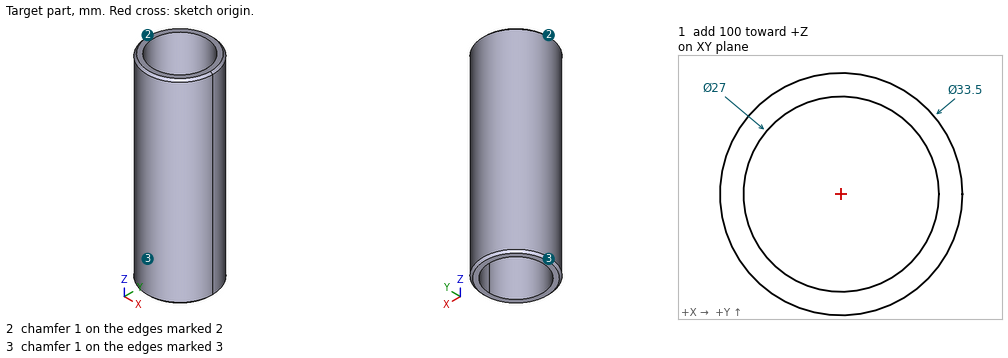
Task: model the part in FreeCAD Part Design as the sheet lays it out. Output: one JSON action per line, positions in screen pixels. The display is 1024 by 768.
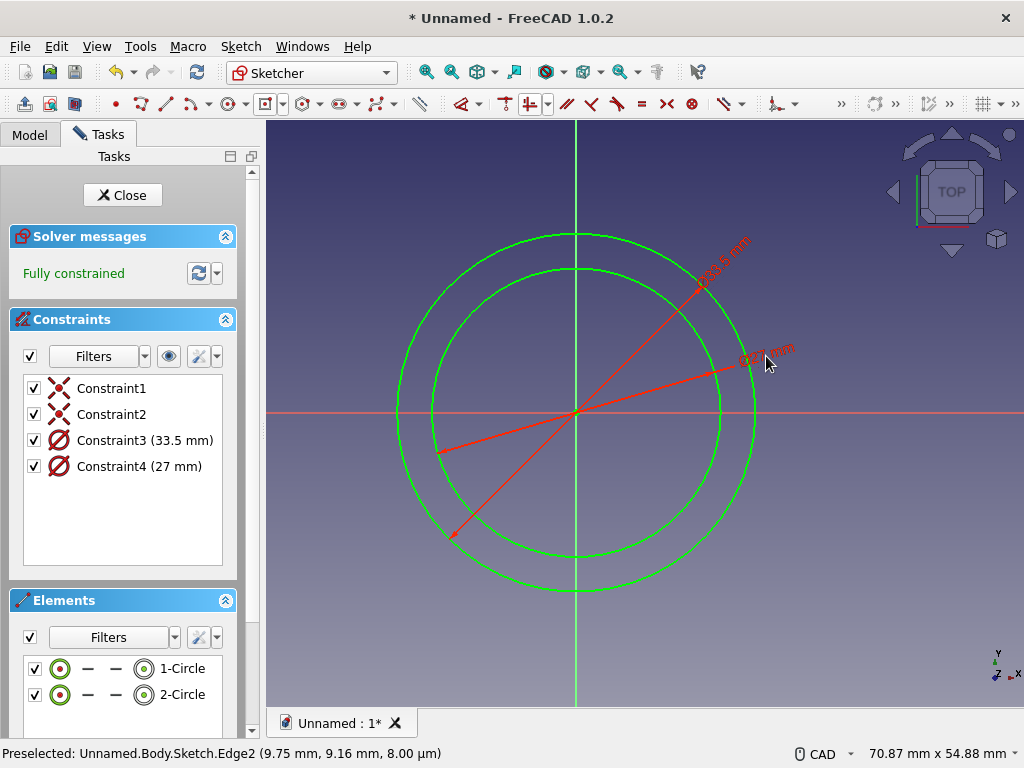
{"action": "left_click", "coordinate": [123, 195]}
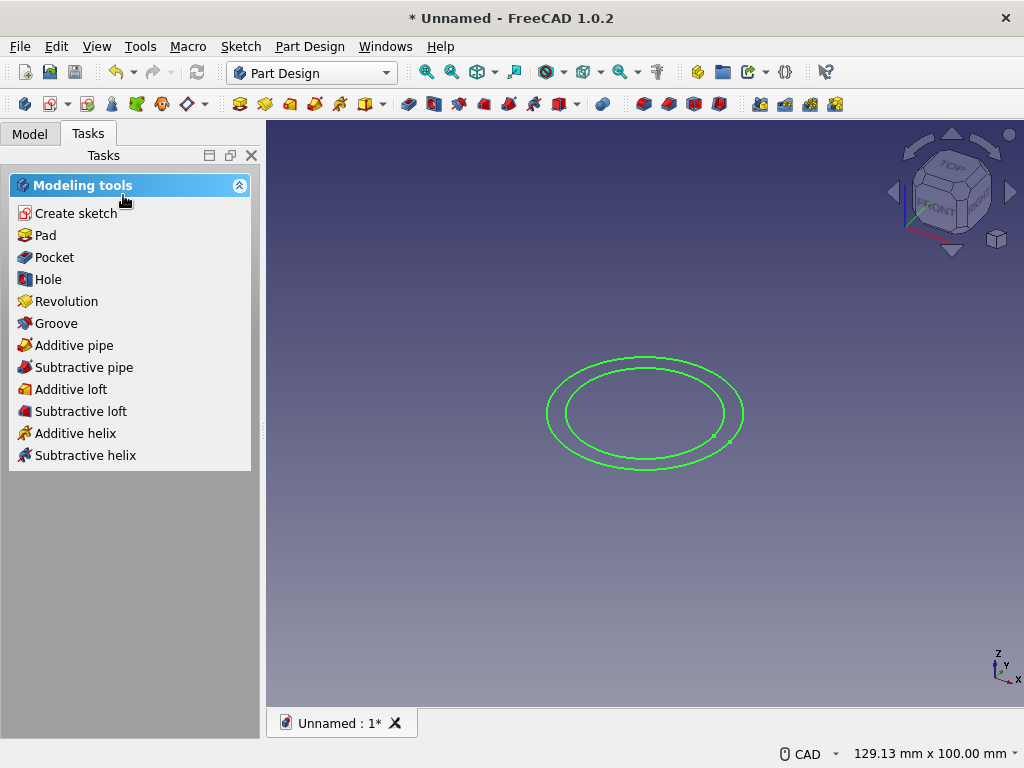
{"action": "left_click", "coordinate": [240, 104]}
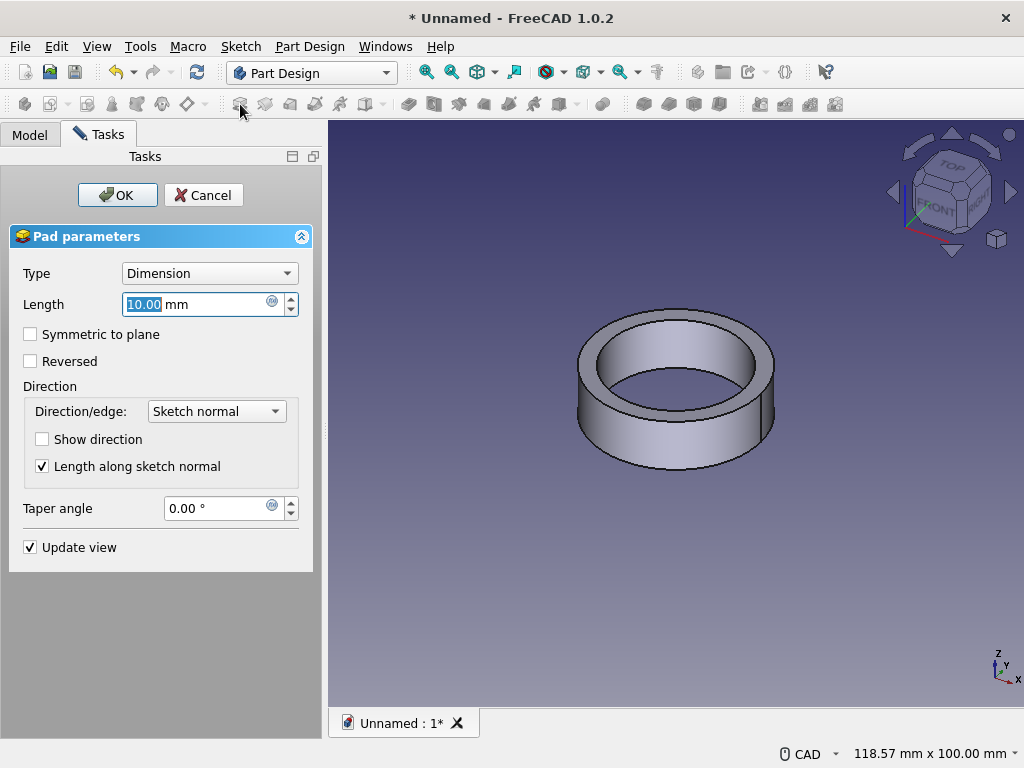
{"action": "type", "text": "100"}
{"action": "key", "text": "Tab"}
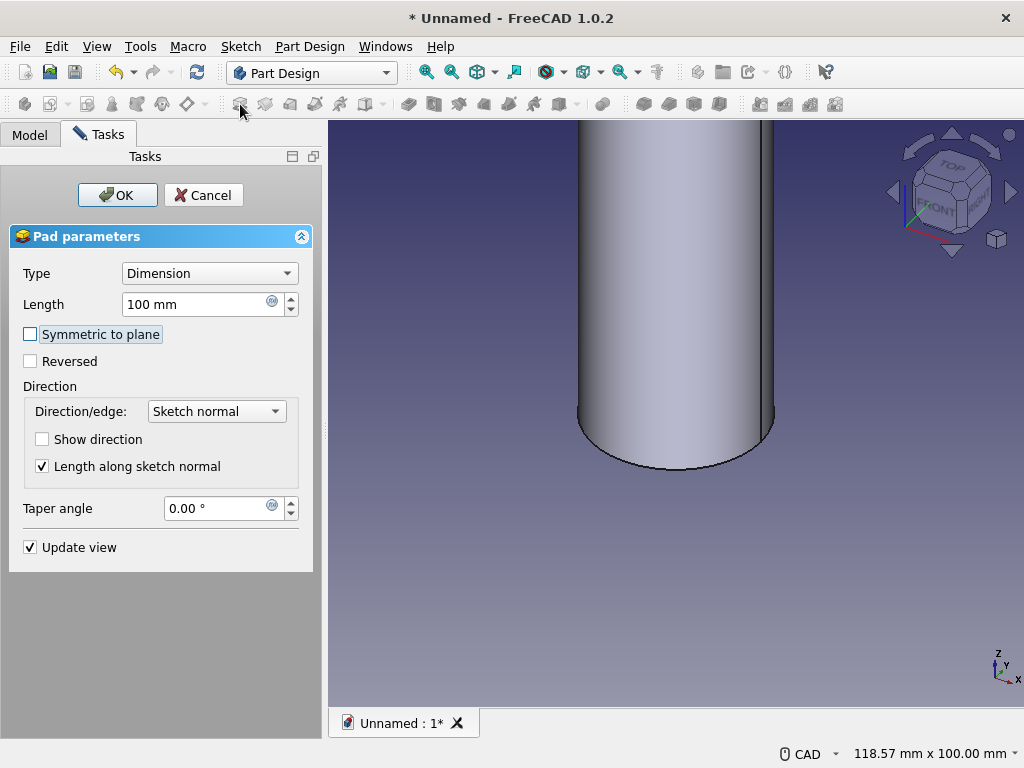
{"action": "left_click", "coordinate": [118, 195]}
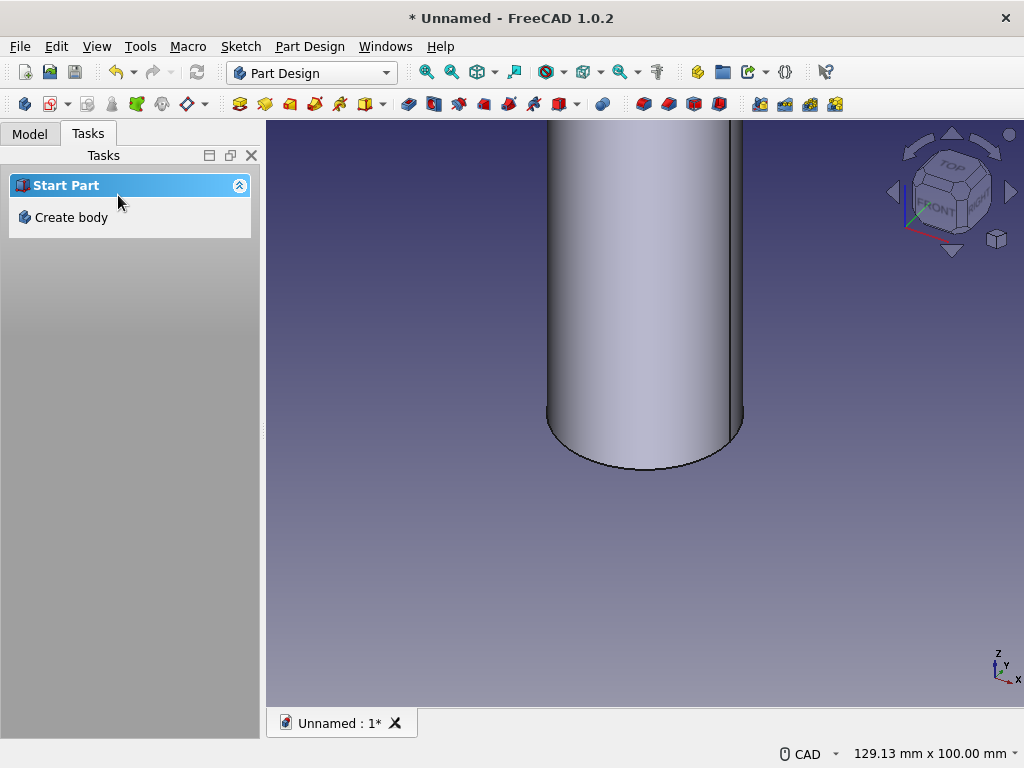
{"action": "left_click", "coordinate": [427, 72]}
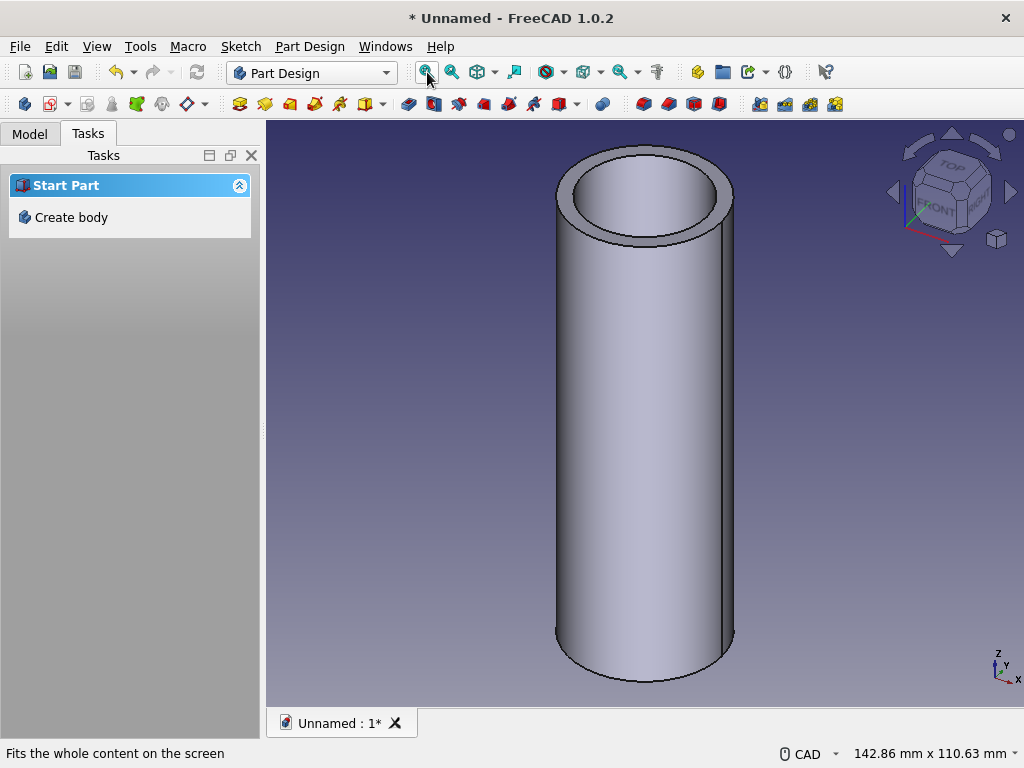
{"action": "left_click", "coordinate": [556, 200]}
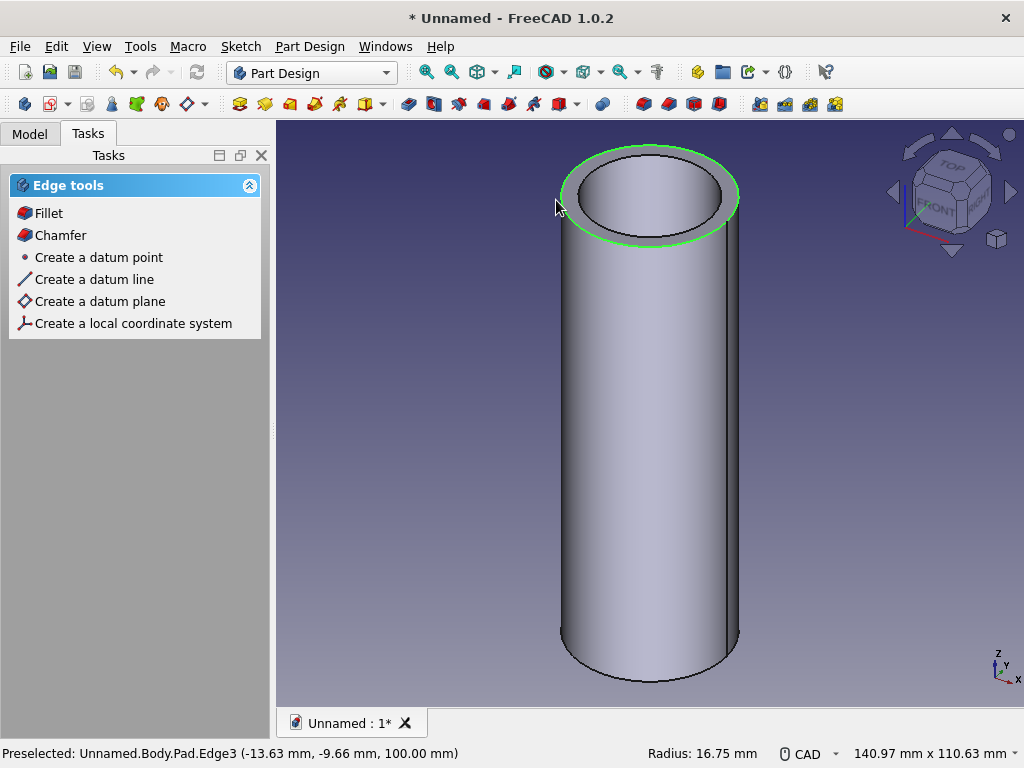
{"action": "left_click", "coordinate": [669, 104]}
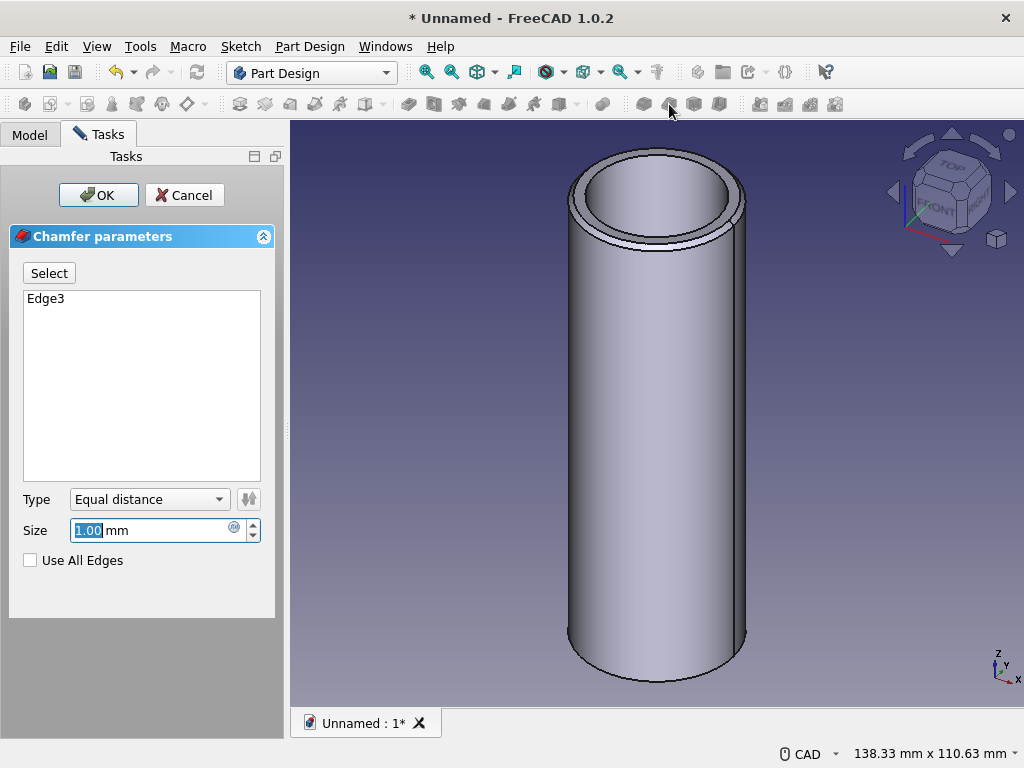
{"action": "type", "text": "1"}
{"action": "key", "text": "Tab"}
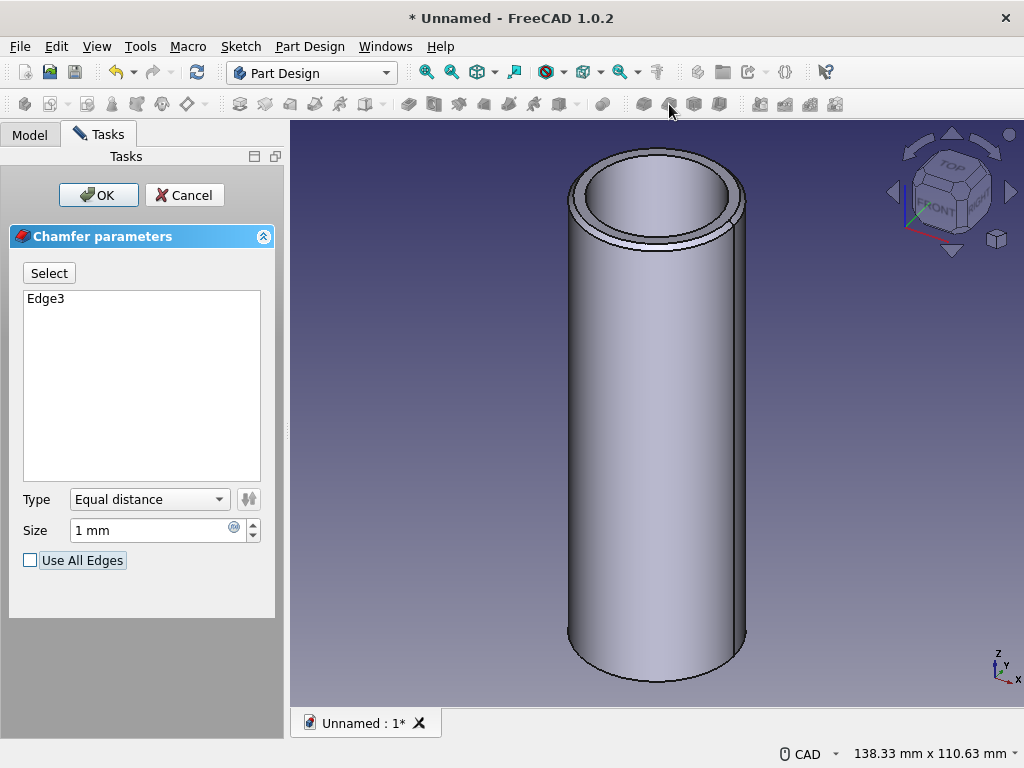
{"action": "left_click", "coordinate": [99, 195]}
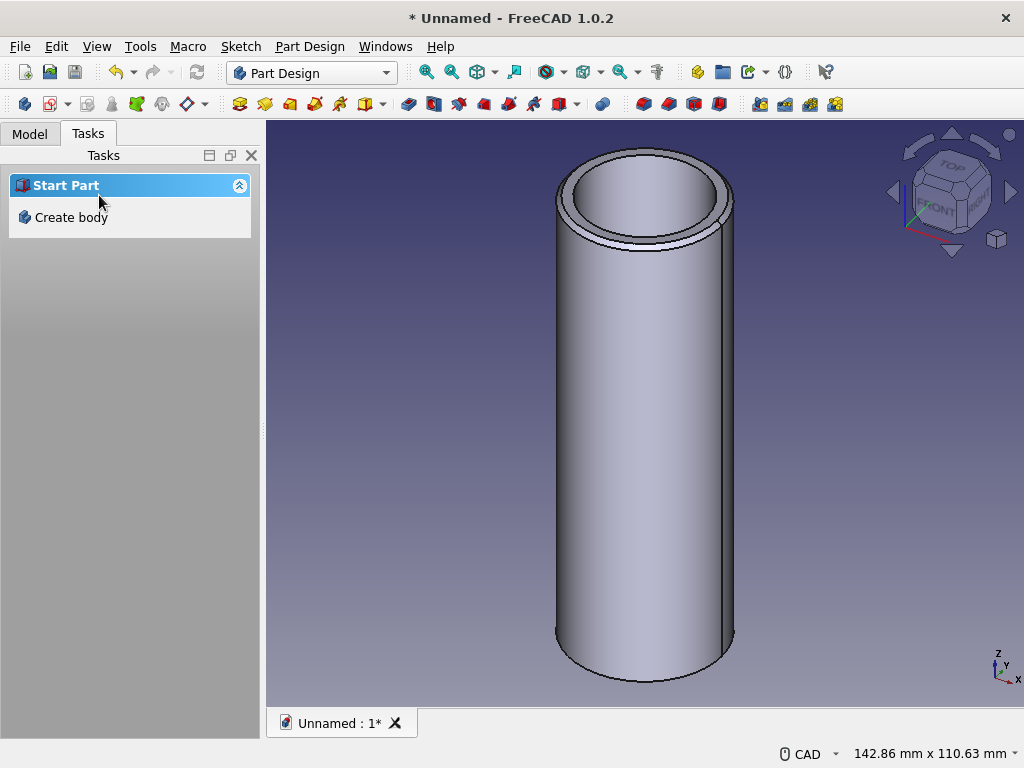
{"action": "key", "text": "0"}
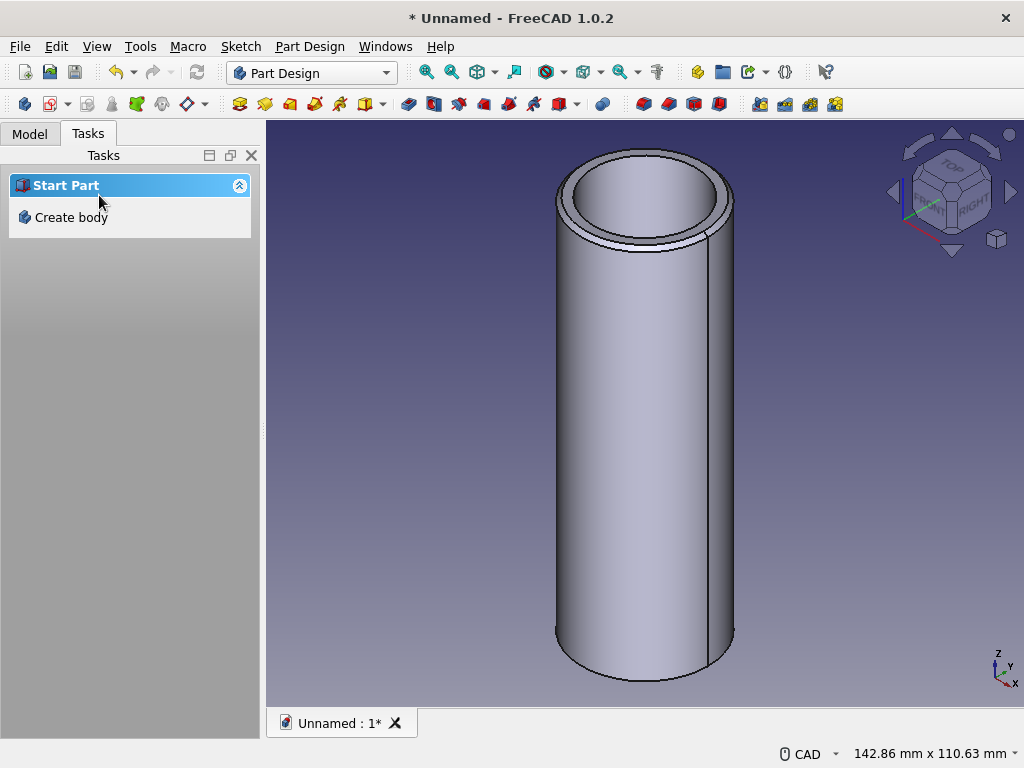
{"action": "key", "text": "2"}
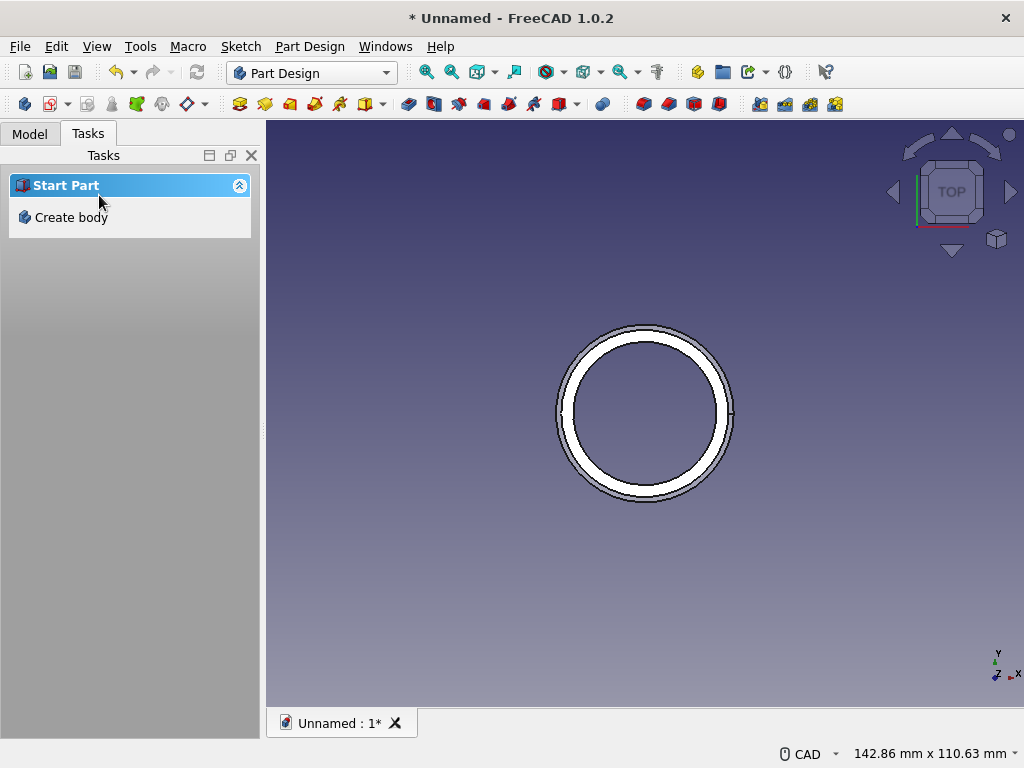
{"action": "left_click", "coordinate": [427, 72]}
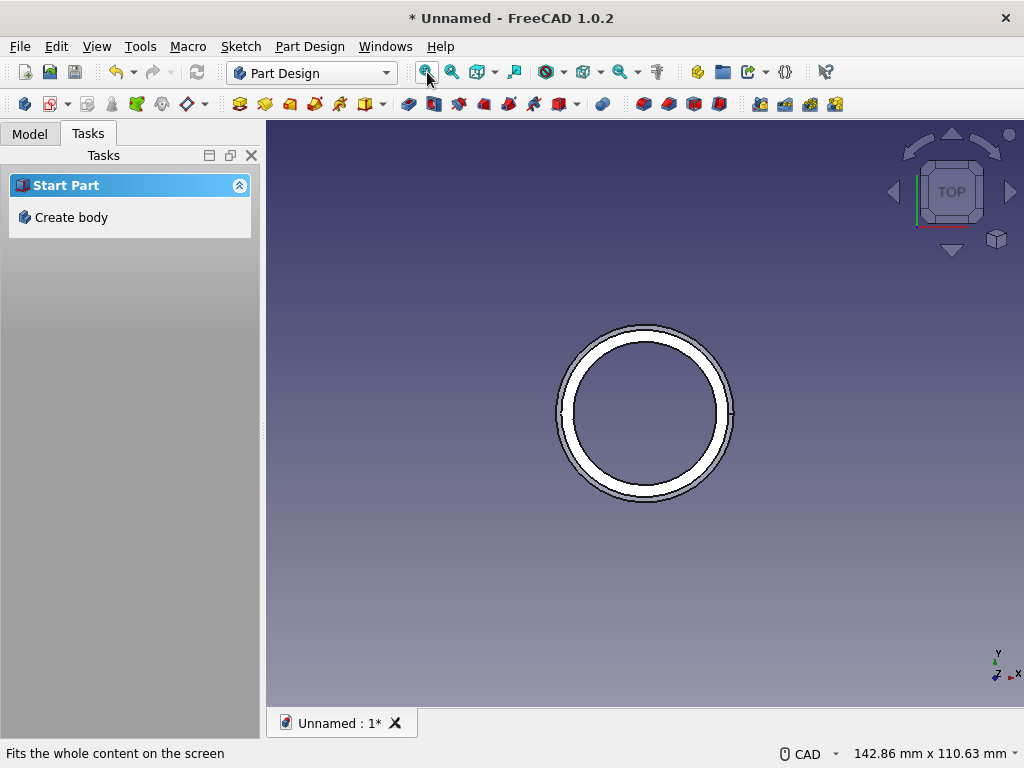
{"action": "key", "text": "1"}